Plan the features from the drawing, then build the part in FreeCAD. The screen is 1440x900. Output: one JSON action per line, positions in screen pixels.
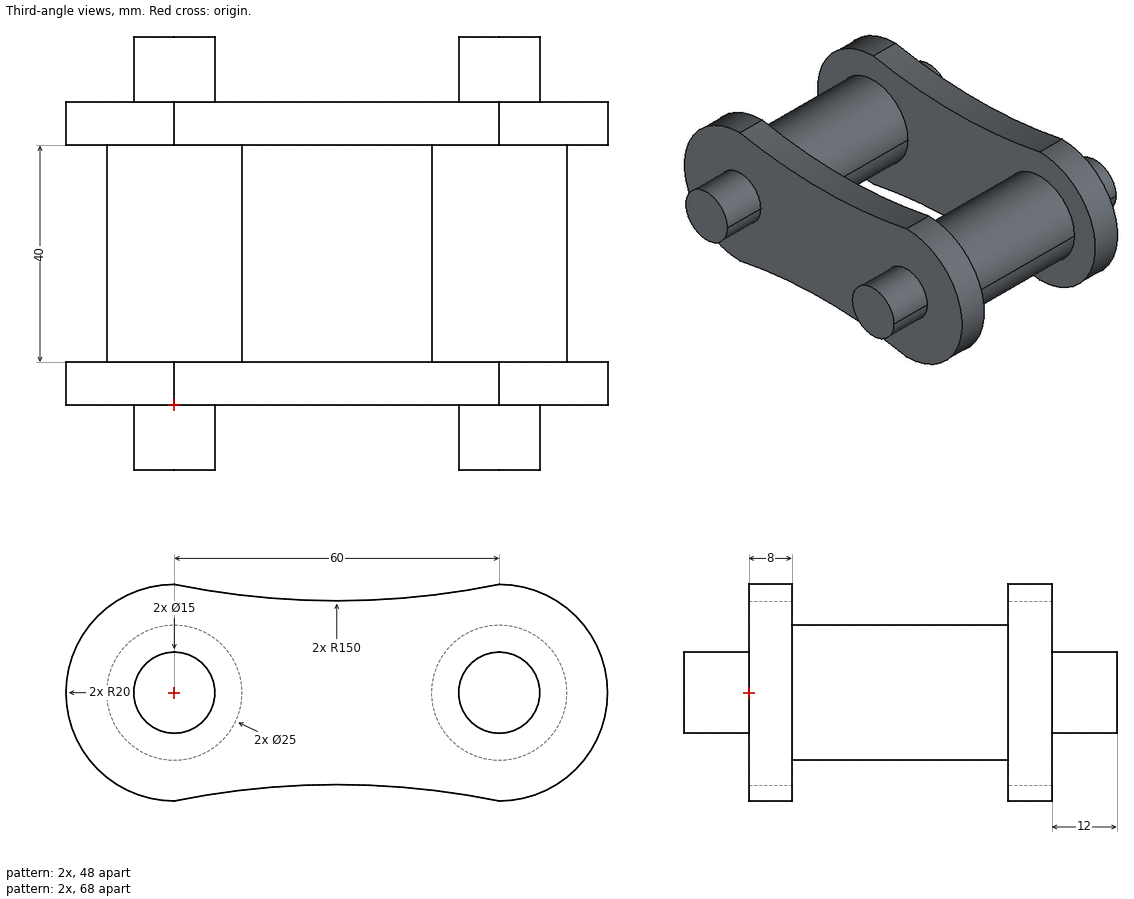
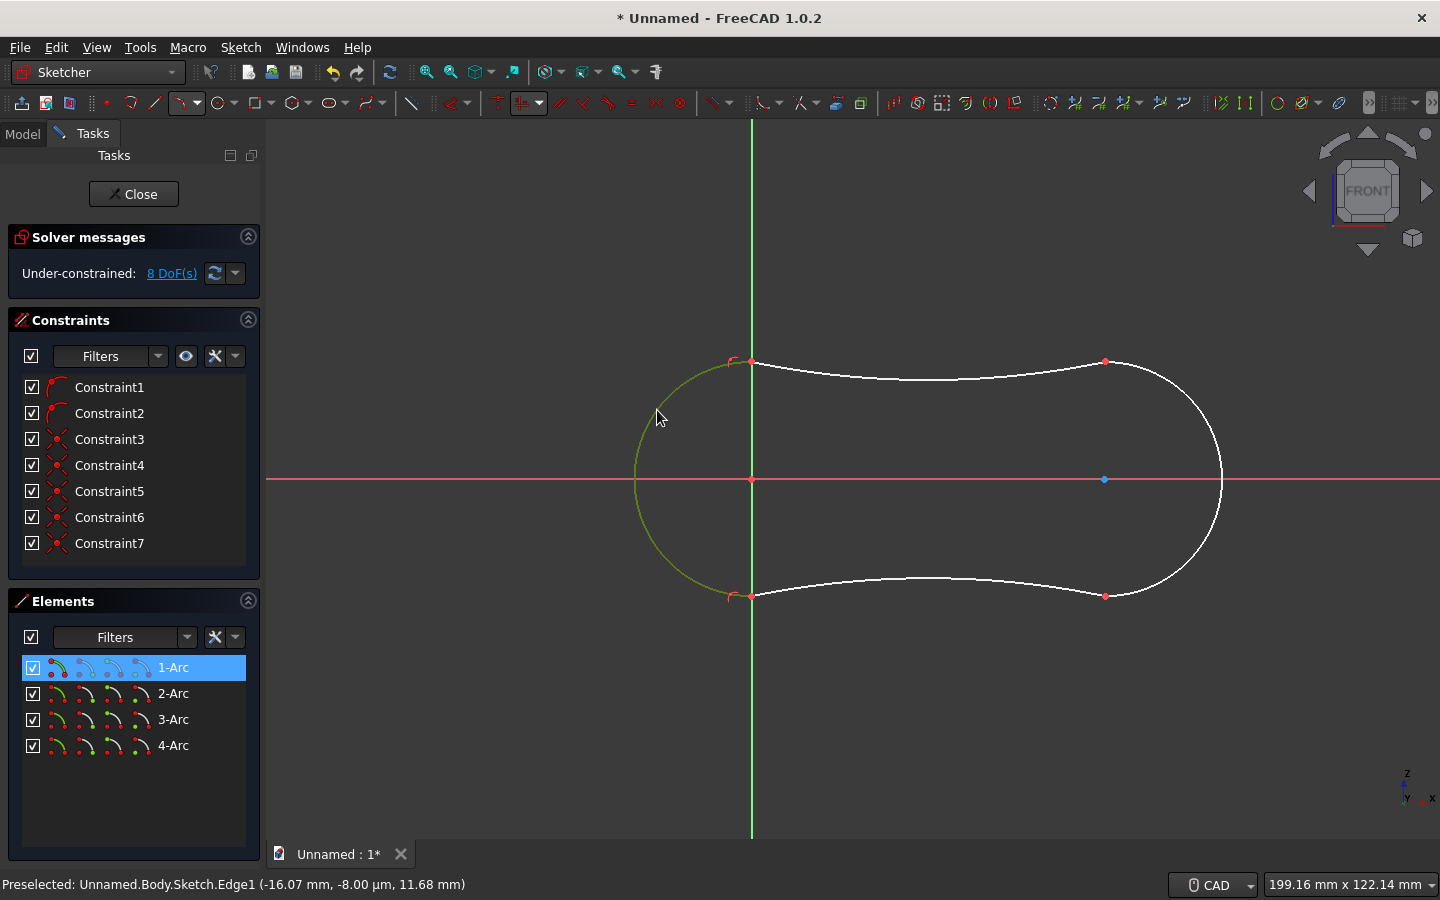
{"action": "left_click", "coordinate": [1200, 548]}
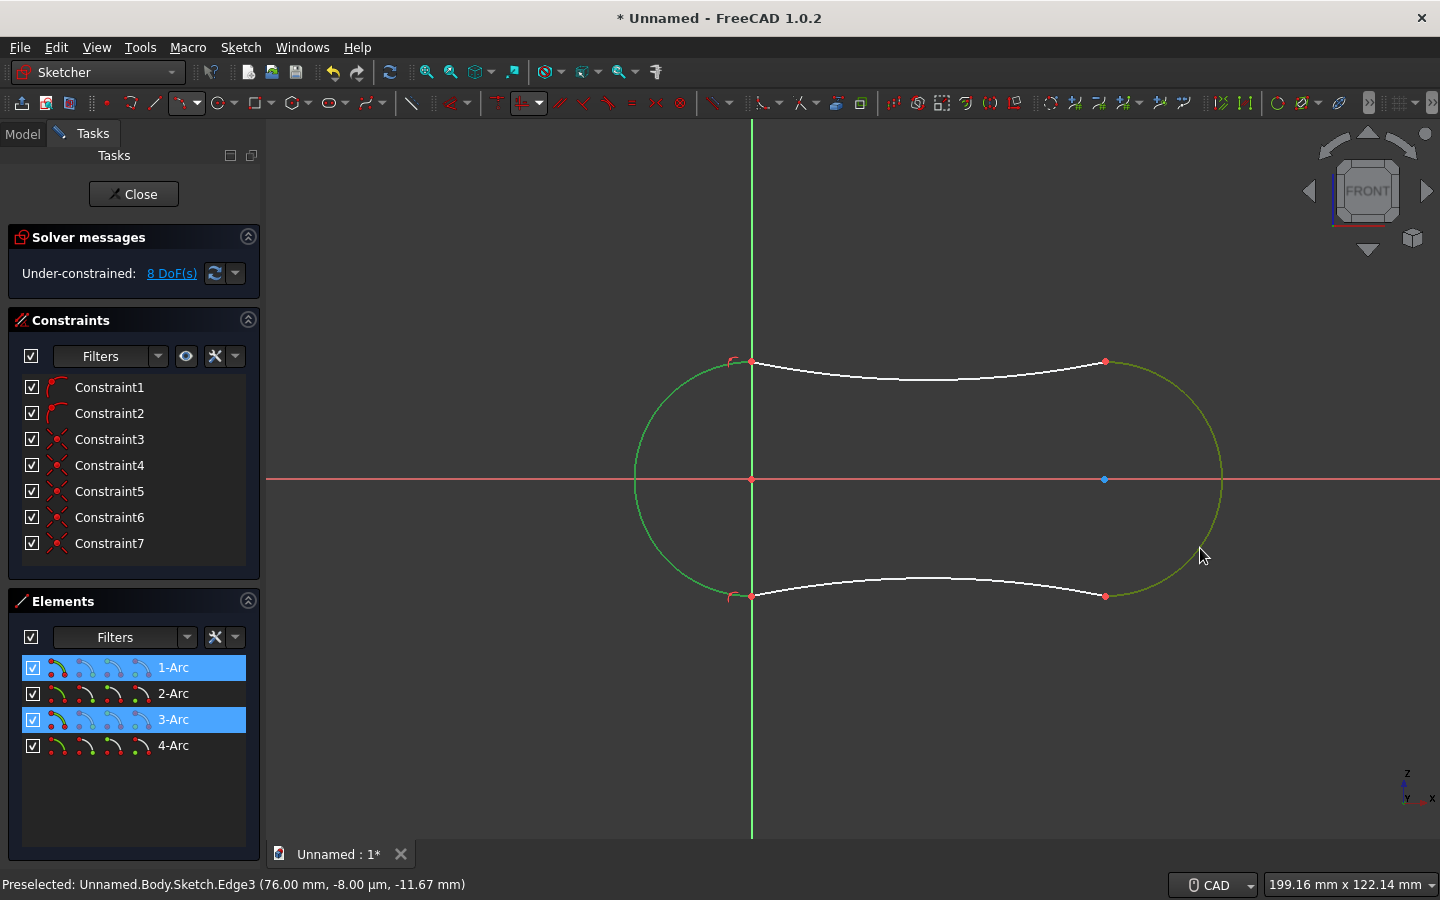
{"action": "left_click", "coordinate": [632, 104]}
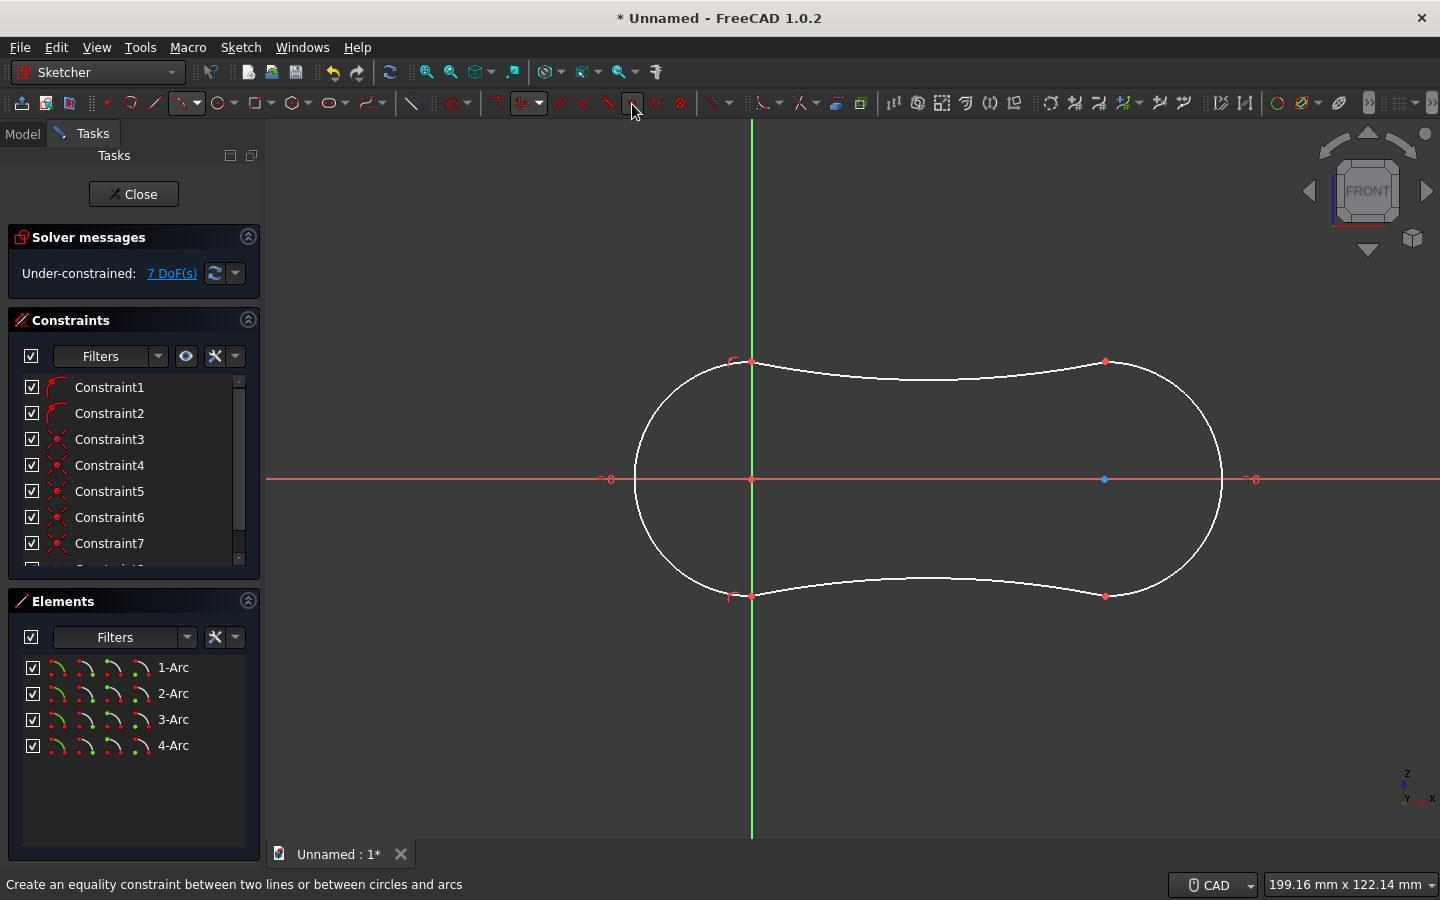
{"action": "left_click", "coordinate": [857, 377]}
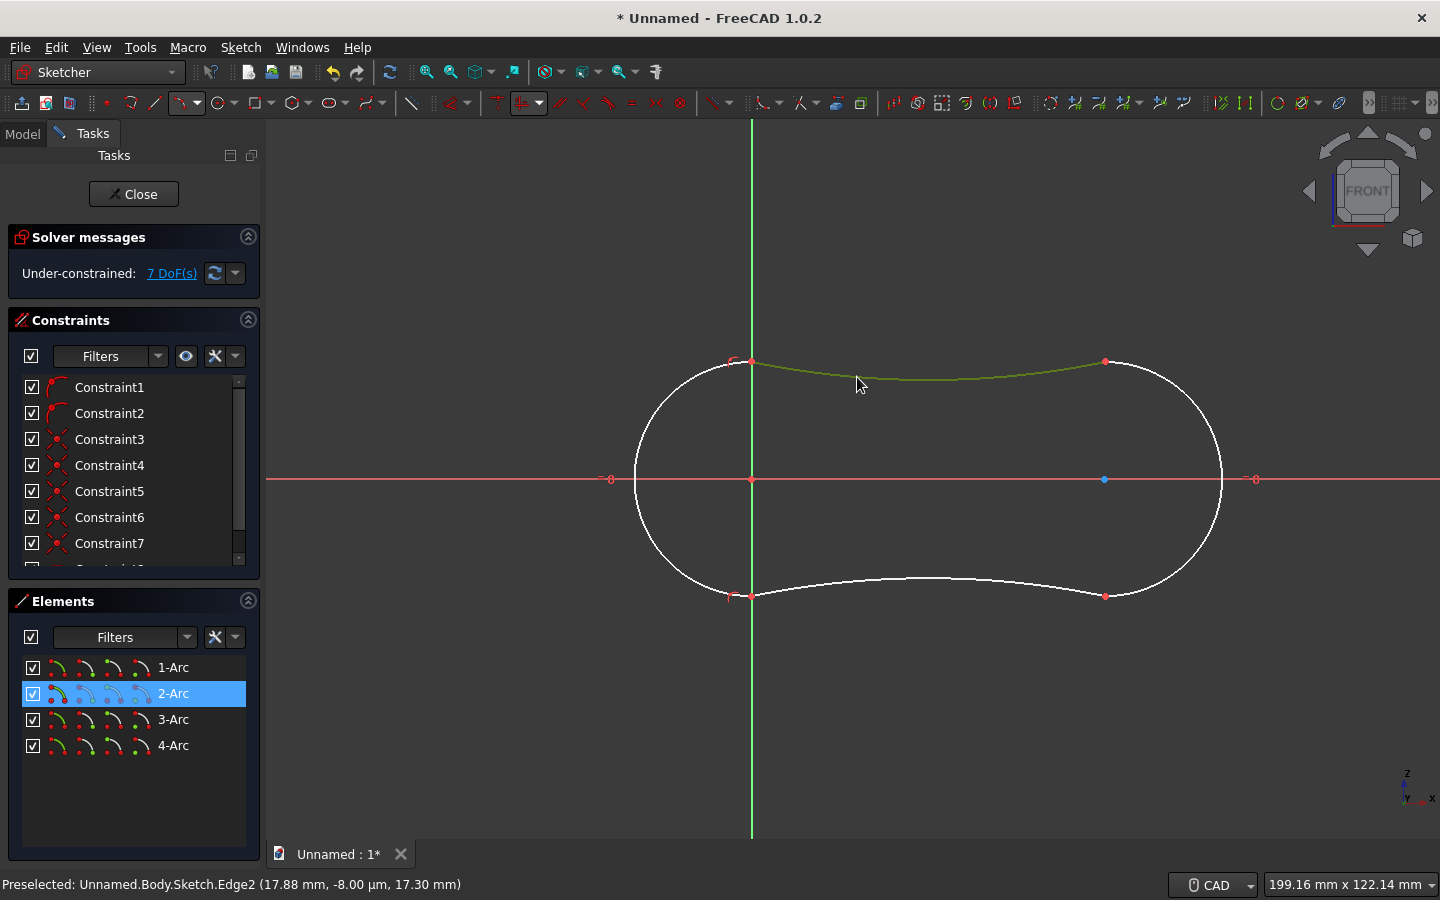
{"action": "left_click", "coordinate": [999, 581]}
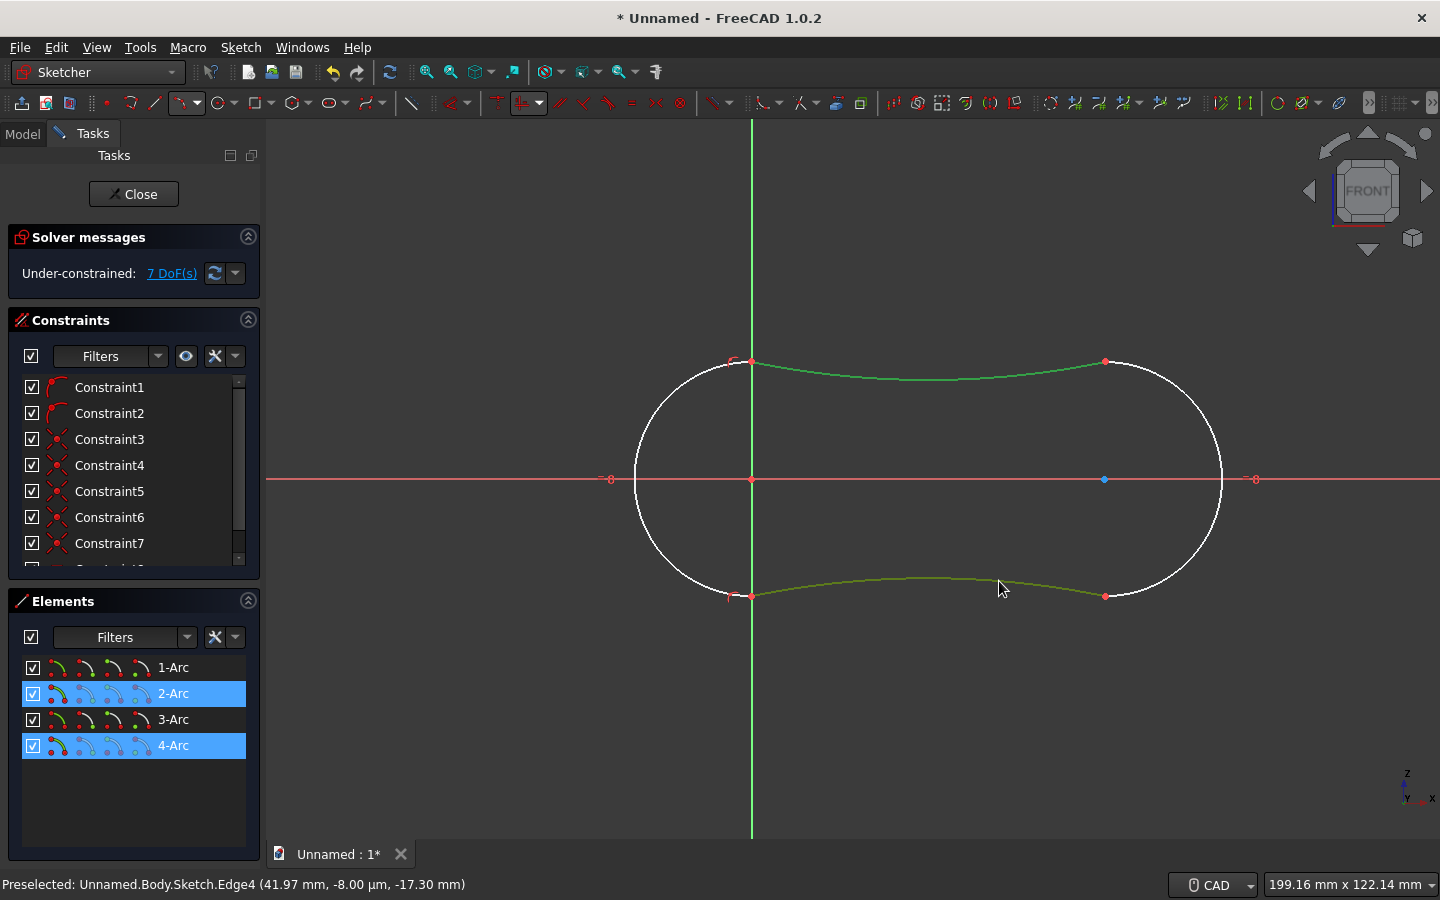
{"action": "left_click", "coordinate": [632, 104]}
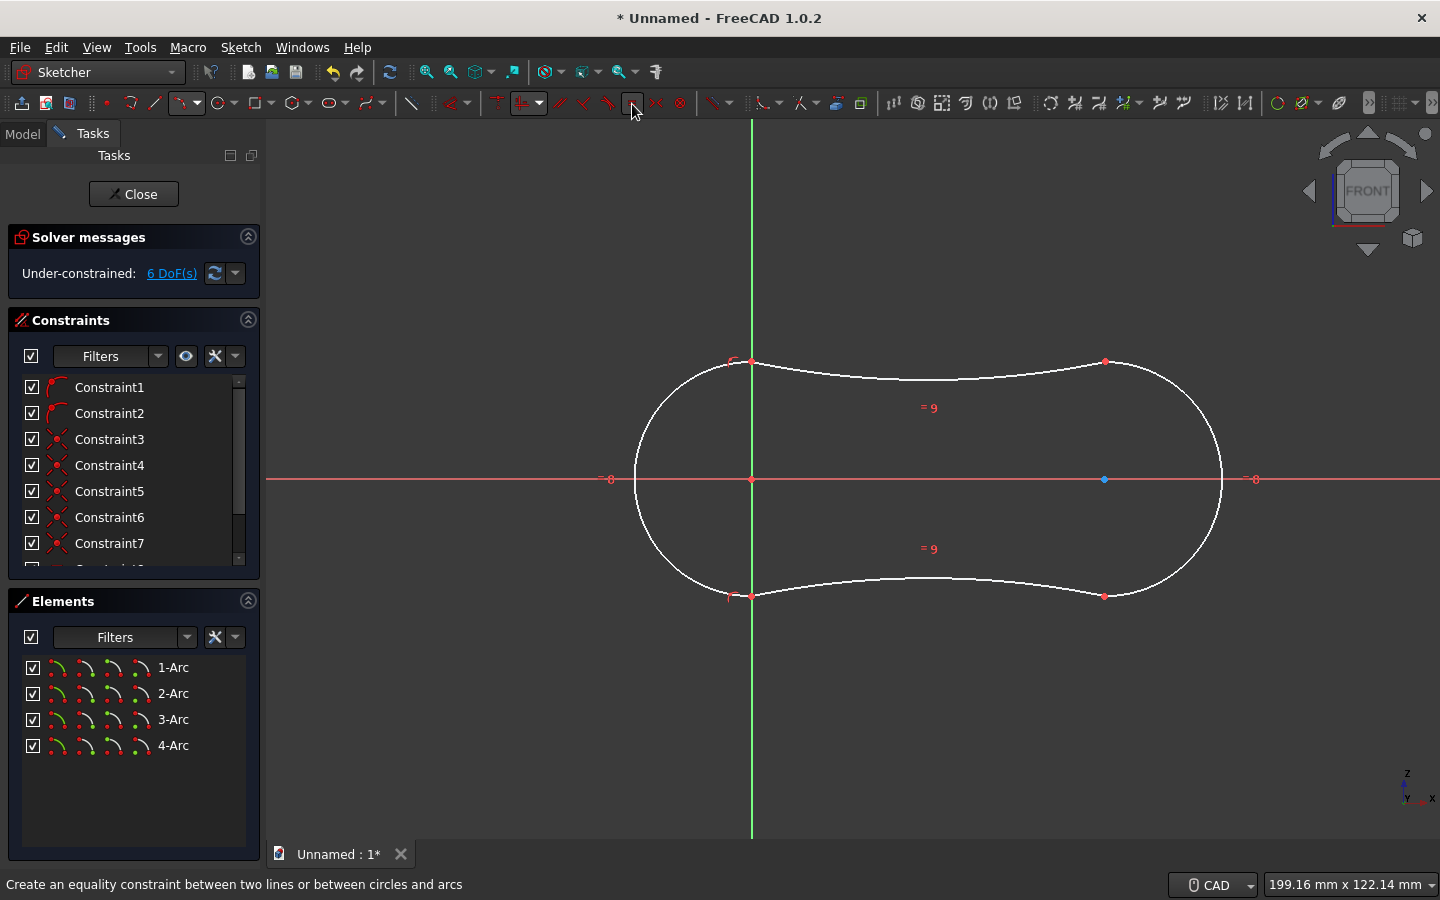
{"action": "left_click", "coordinate": [1105, 479]}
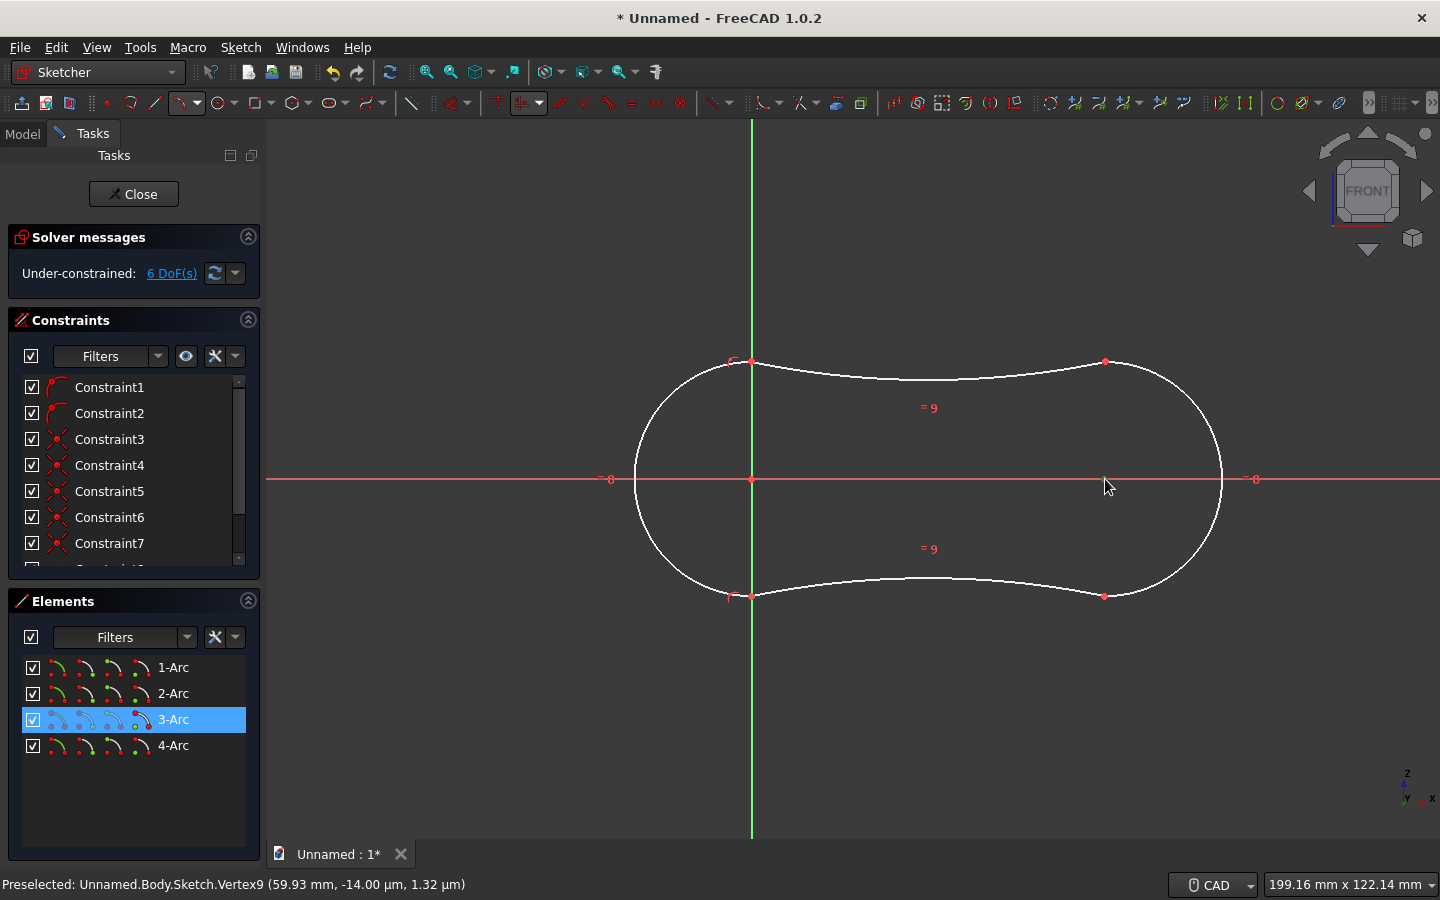
{"action": "left_click", "coordinate": [364, 479]}